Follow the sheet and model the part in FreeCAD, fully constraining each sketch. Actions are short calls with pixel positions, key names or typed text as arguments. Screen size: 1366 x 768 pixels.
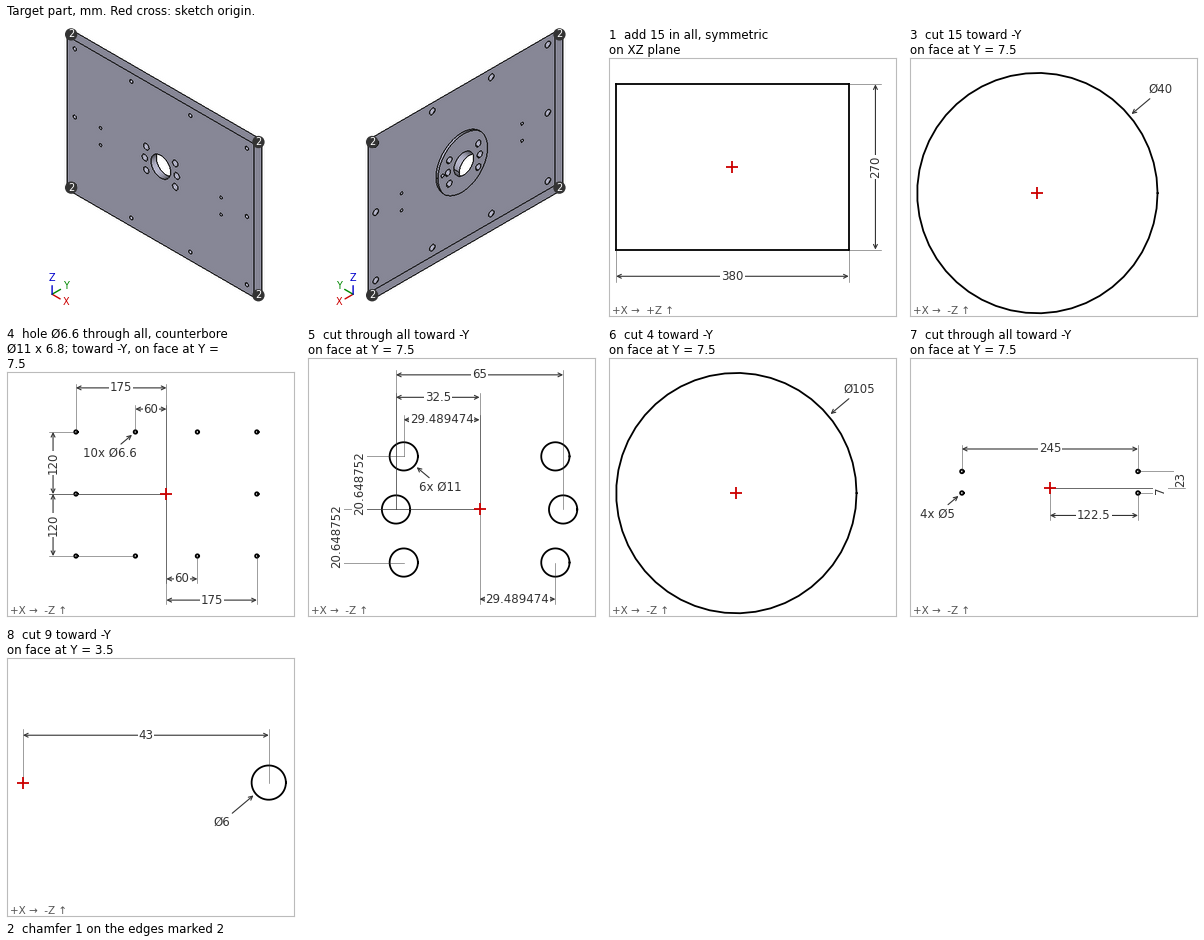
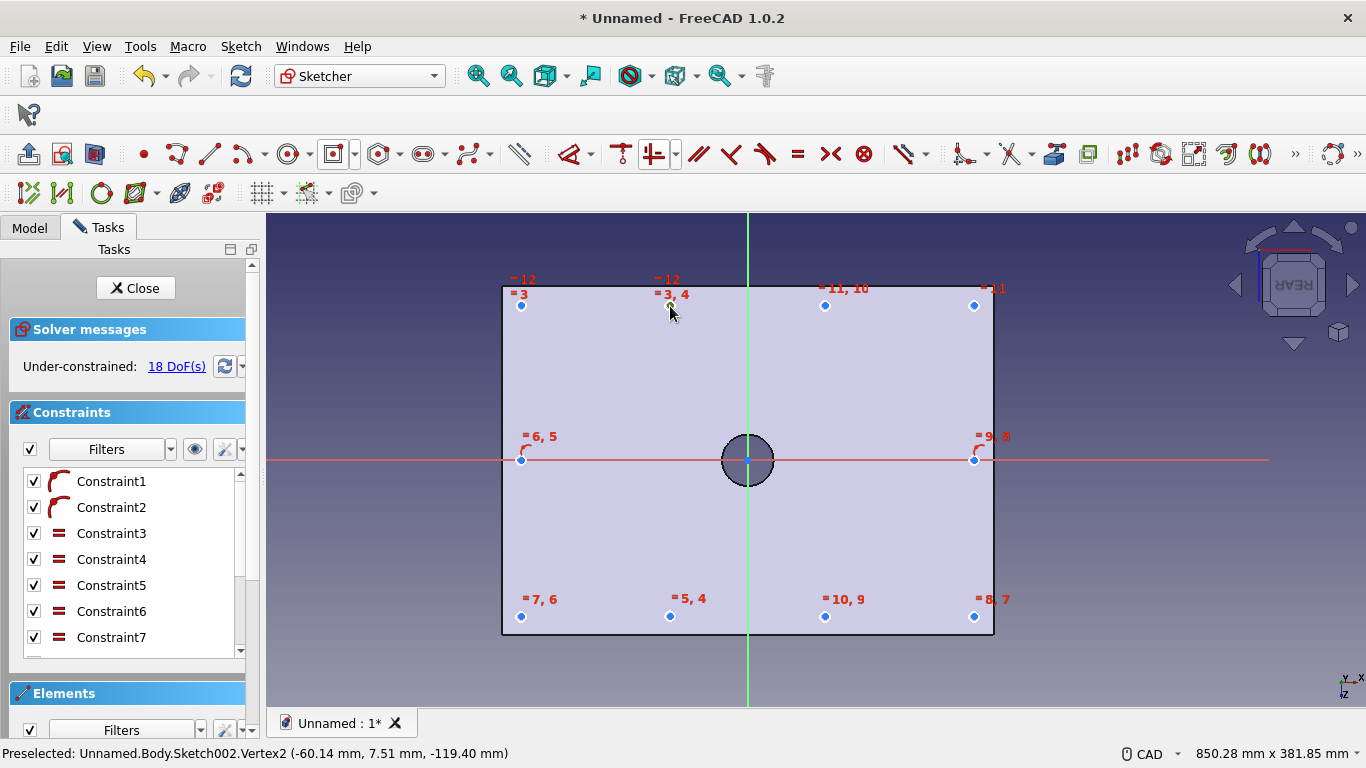
click(670, 616)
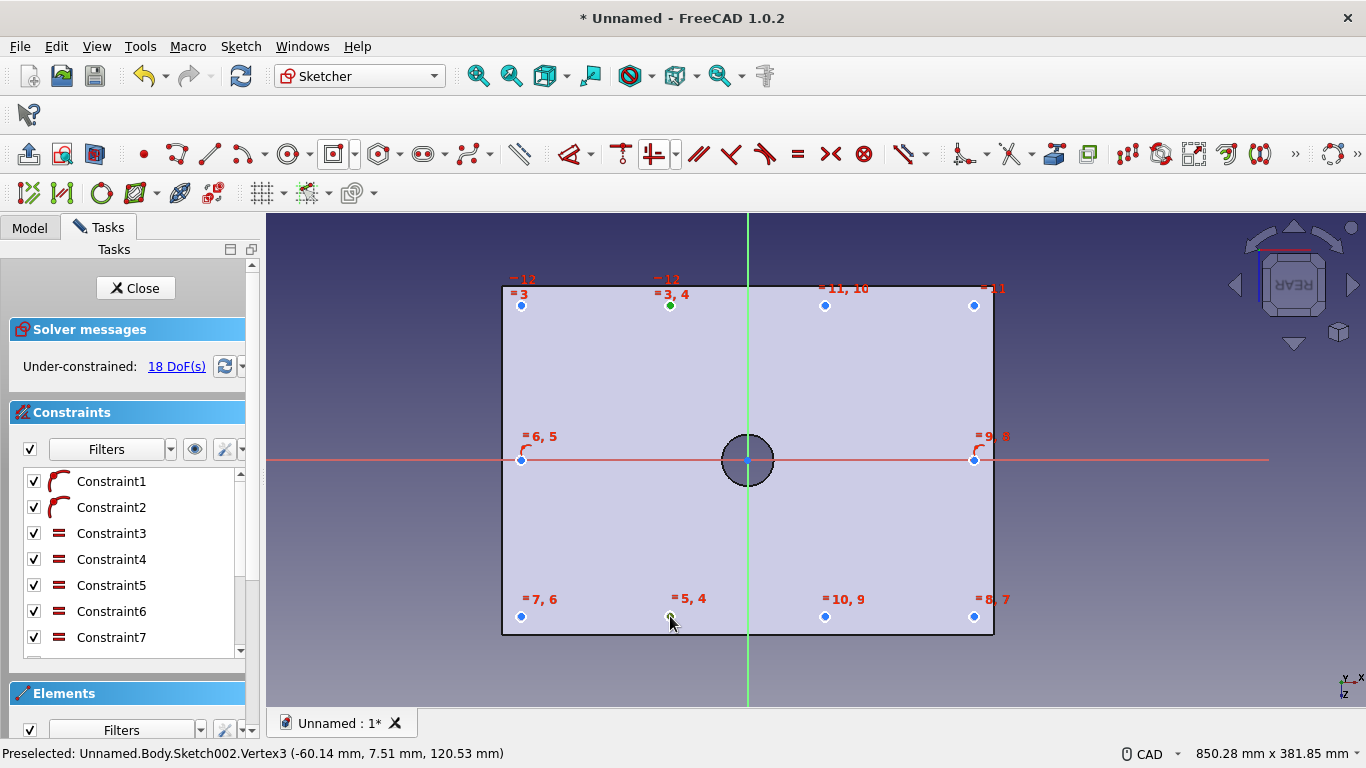
key(v)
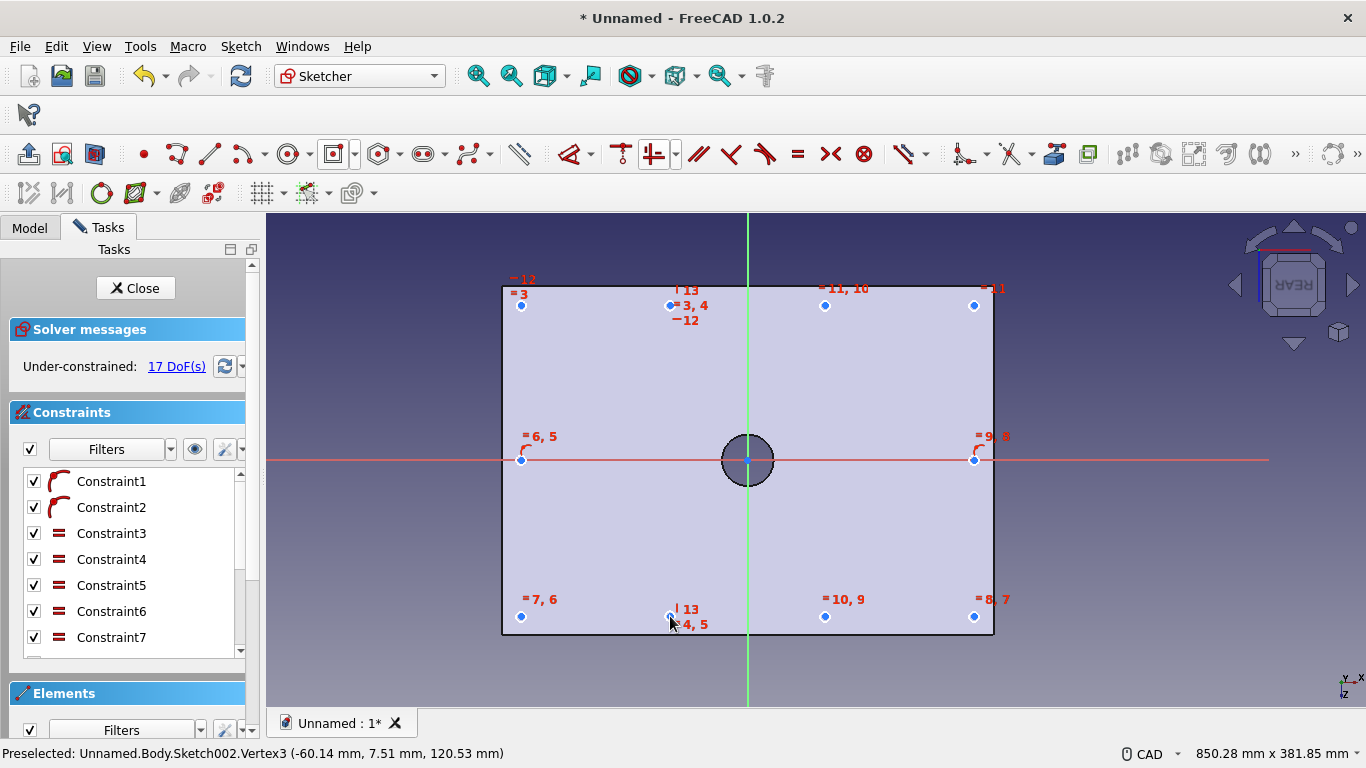
click(521, 306)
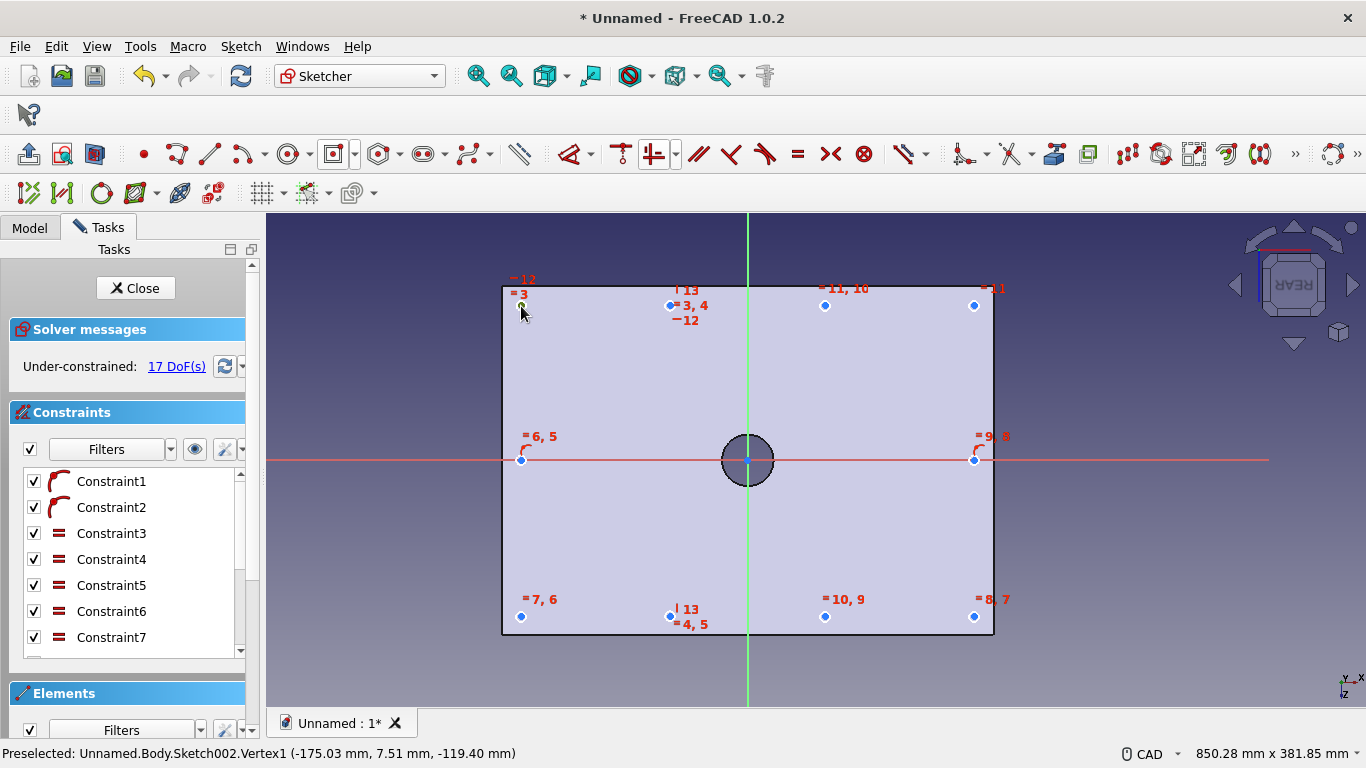
click(521, 460)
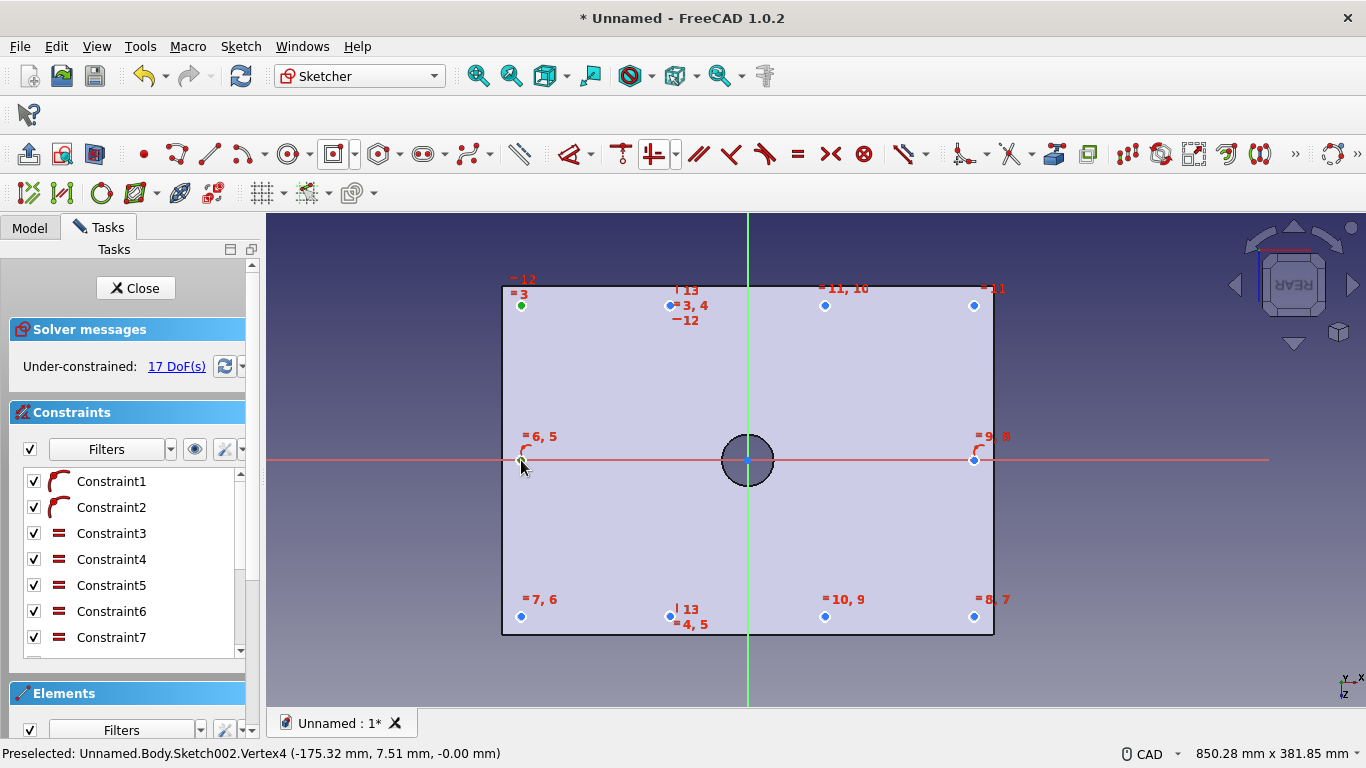
key(v)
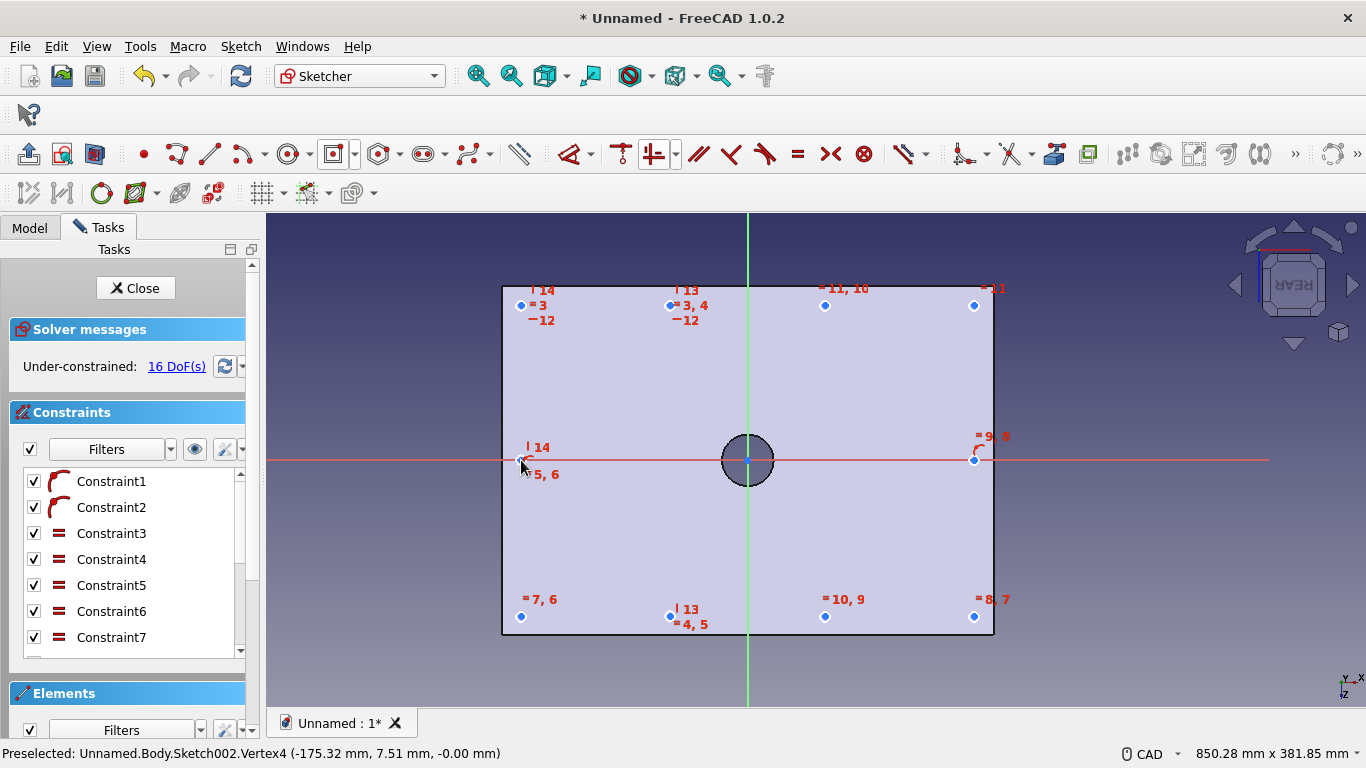
click(521, 460)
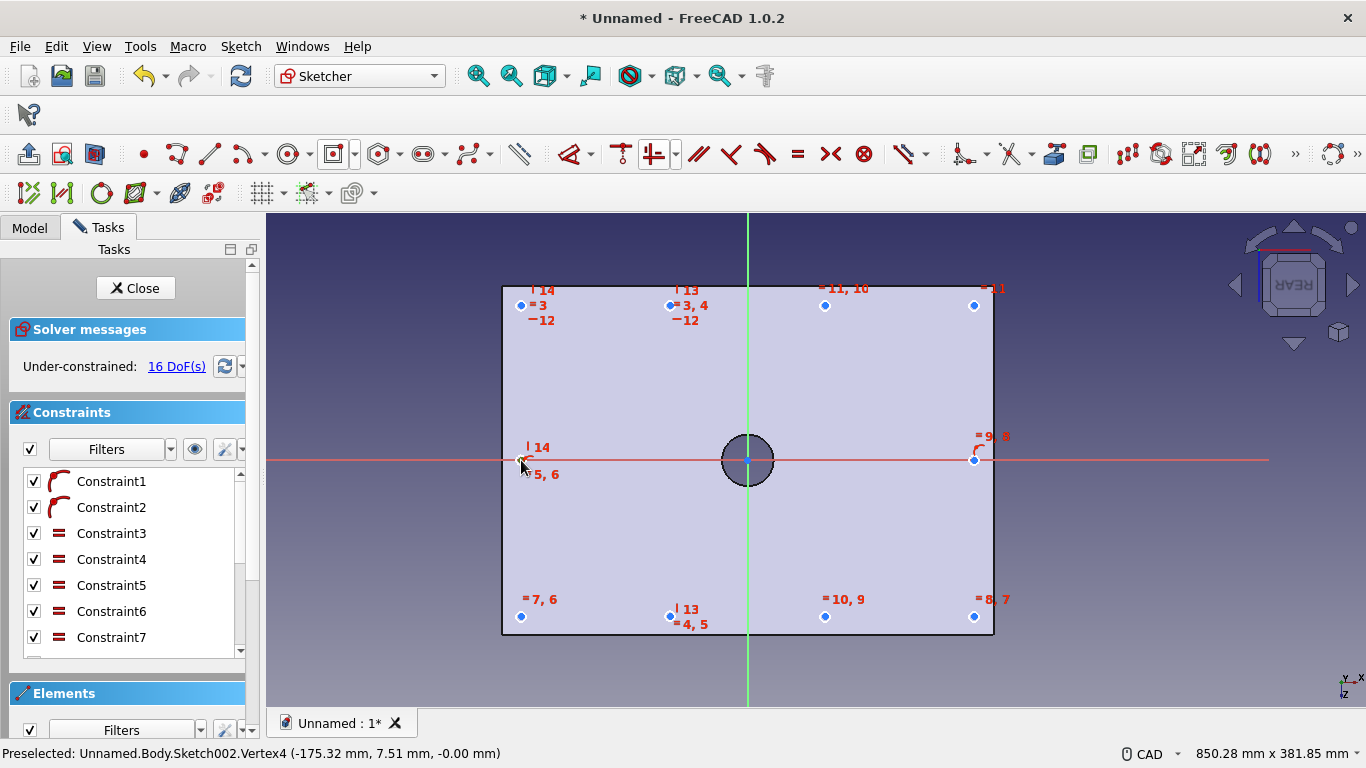
click(521, 617)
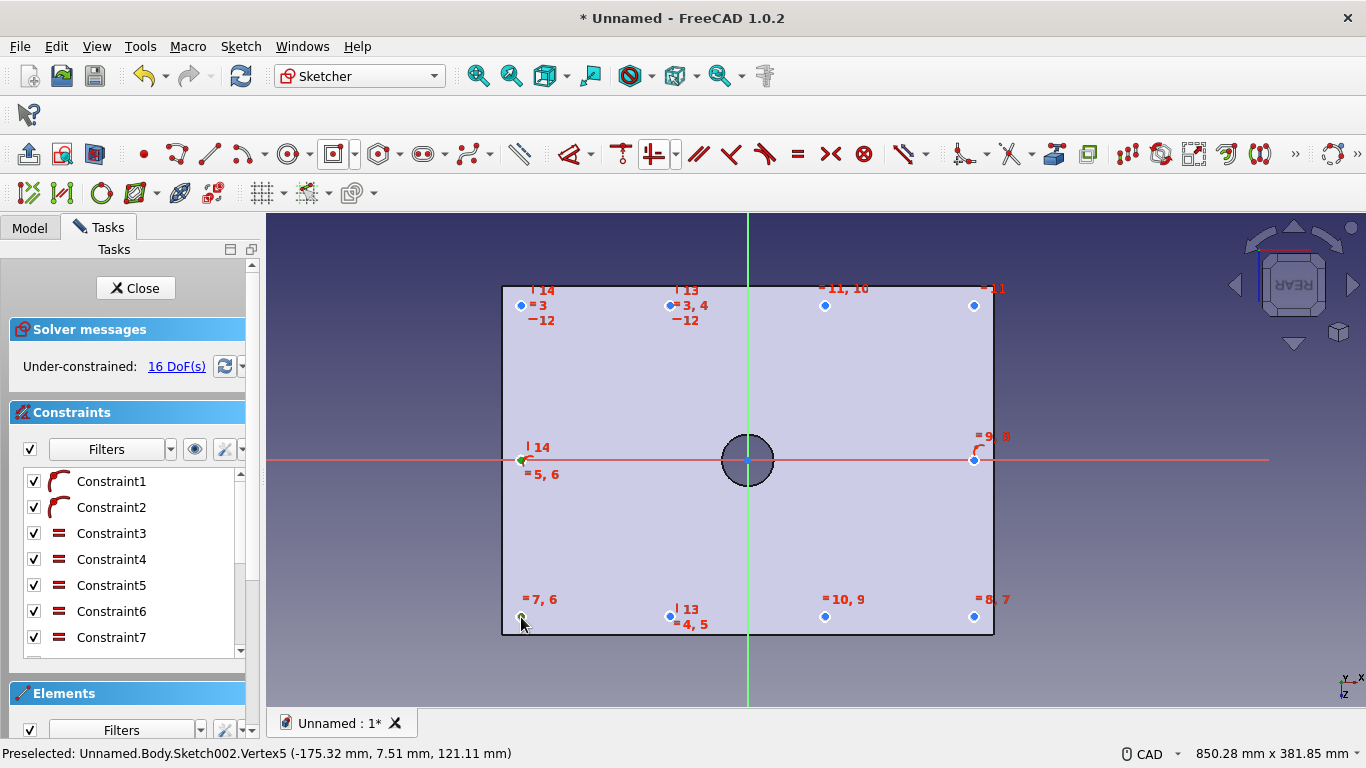
click(676, 154)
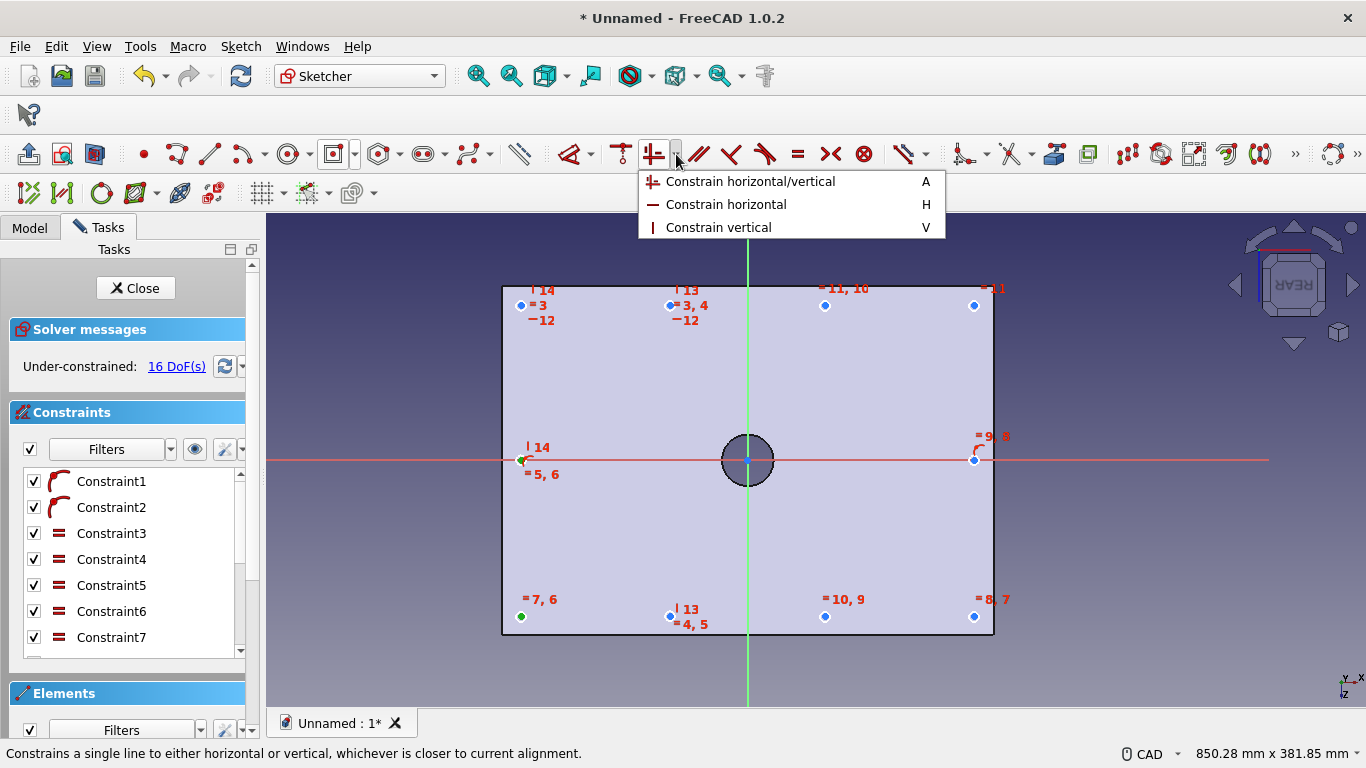
click(792, 228)